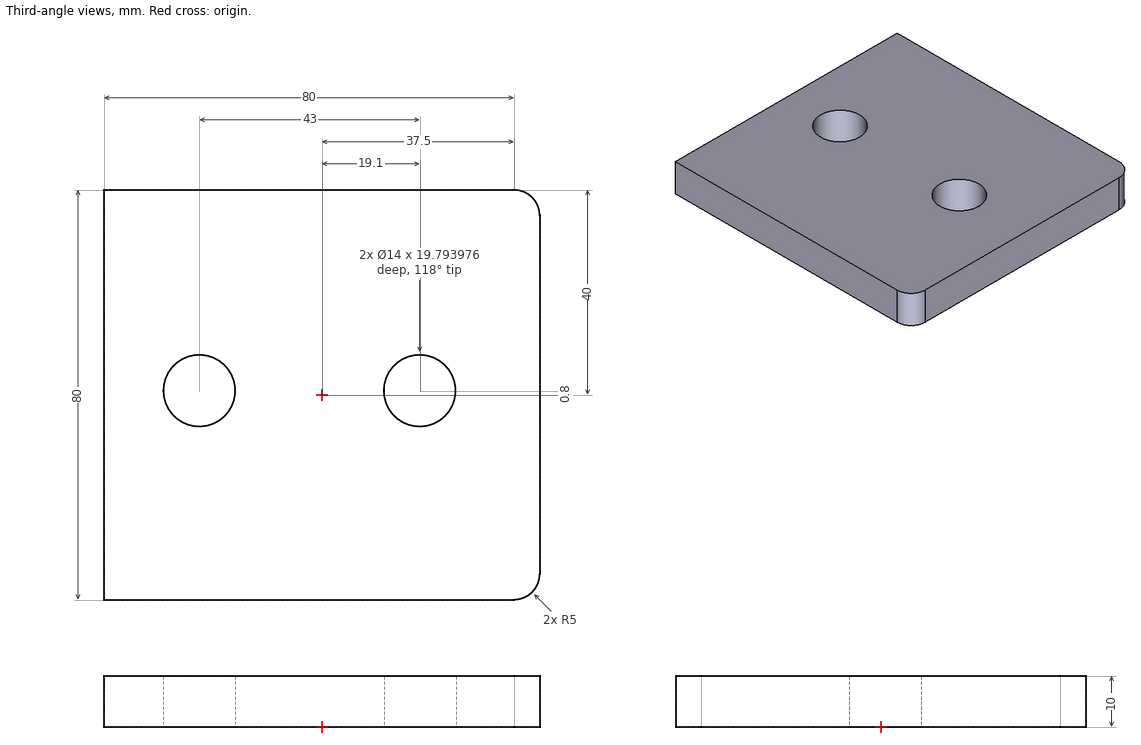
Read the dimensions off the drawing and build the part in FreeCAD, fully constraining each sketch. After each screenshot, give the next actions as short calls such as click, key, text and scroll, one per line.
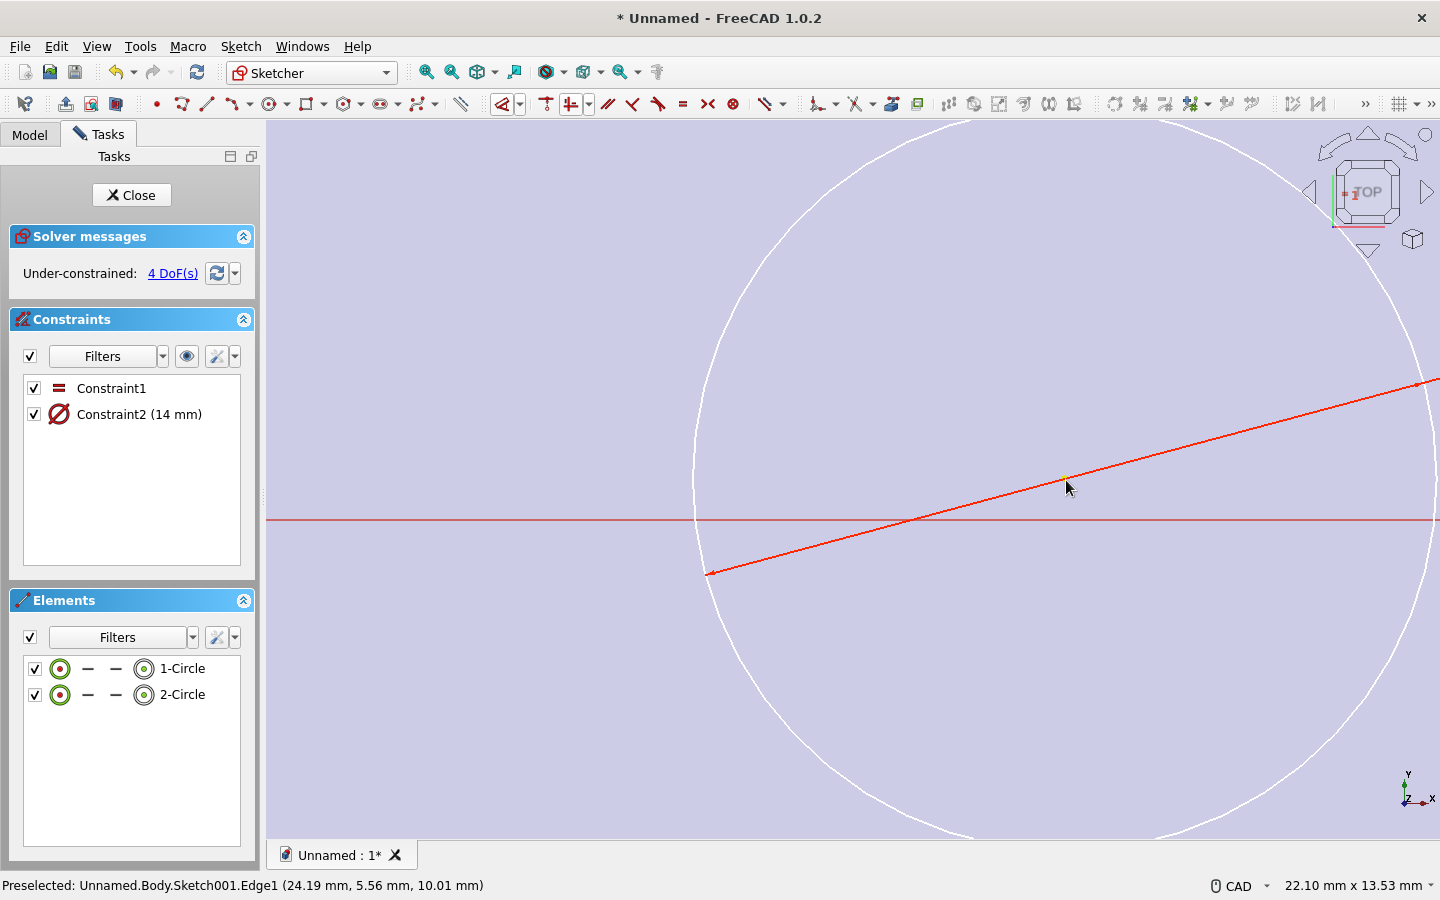
click(1065, 479)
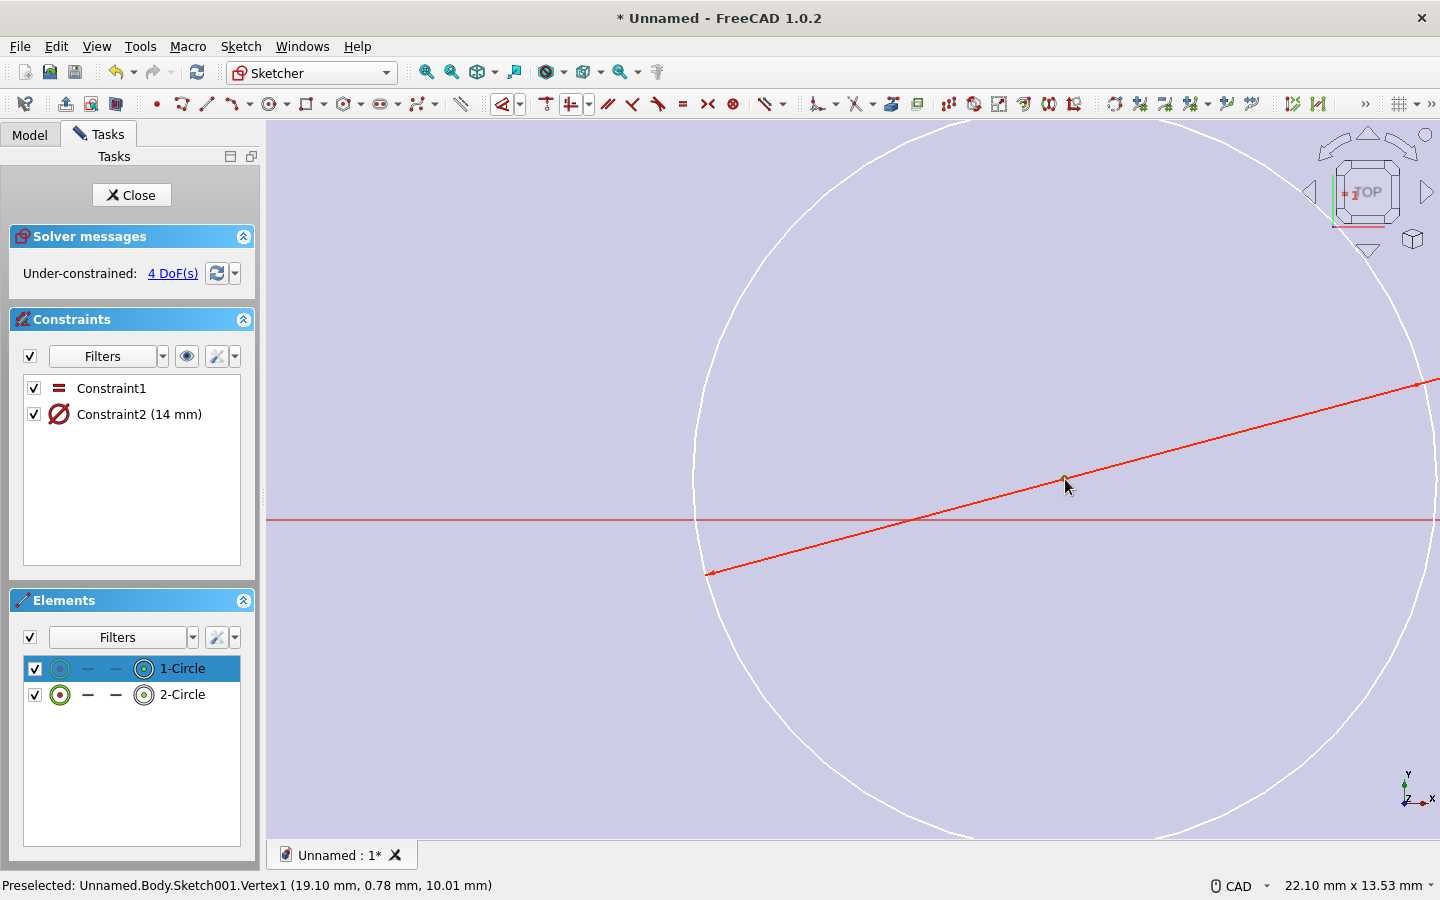
key(i)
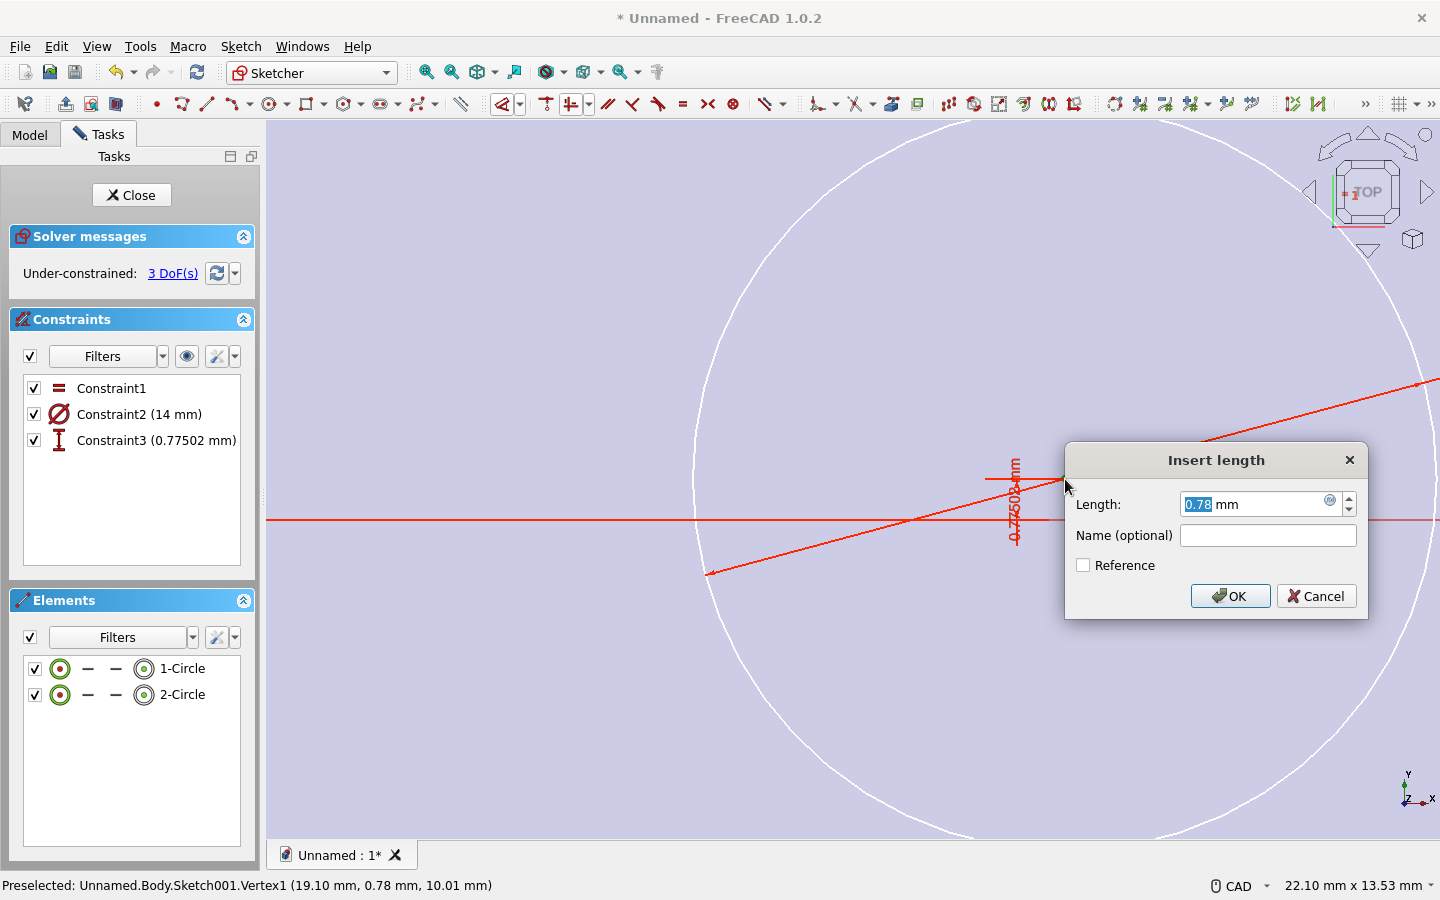
text(0.8)
key(Return)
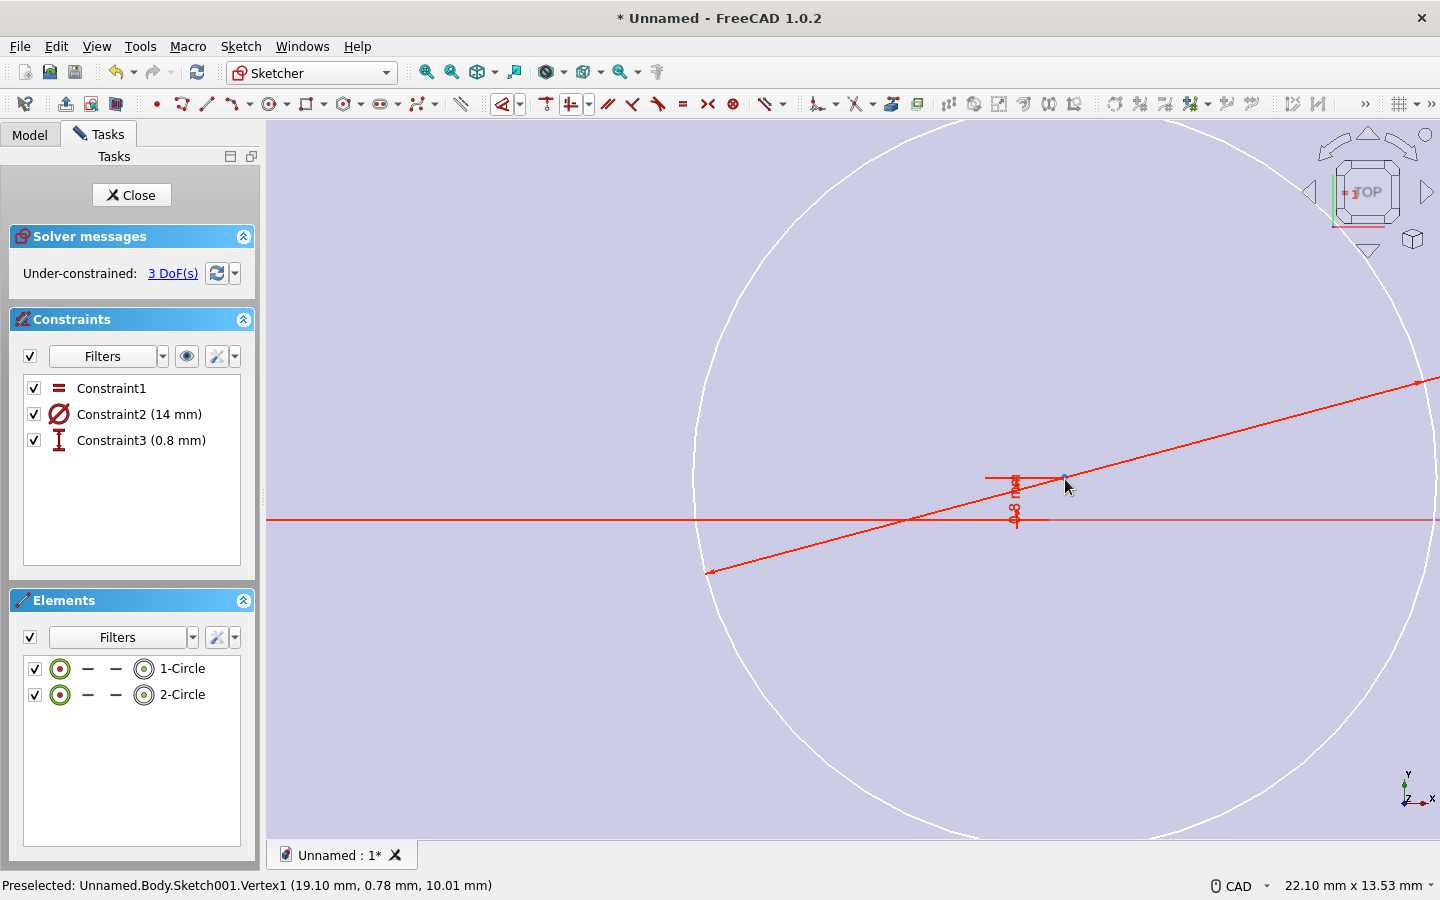
scroll(1067, 480, down, 7)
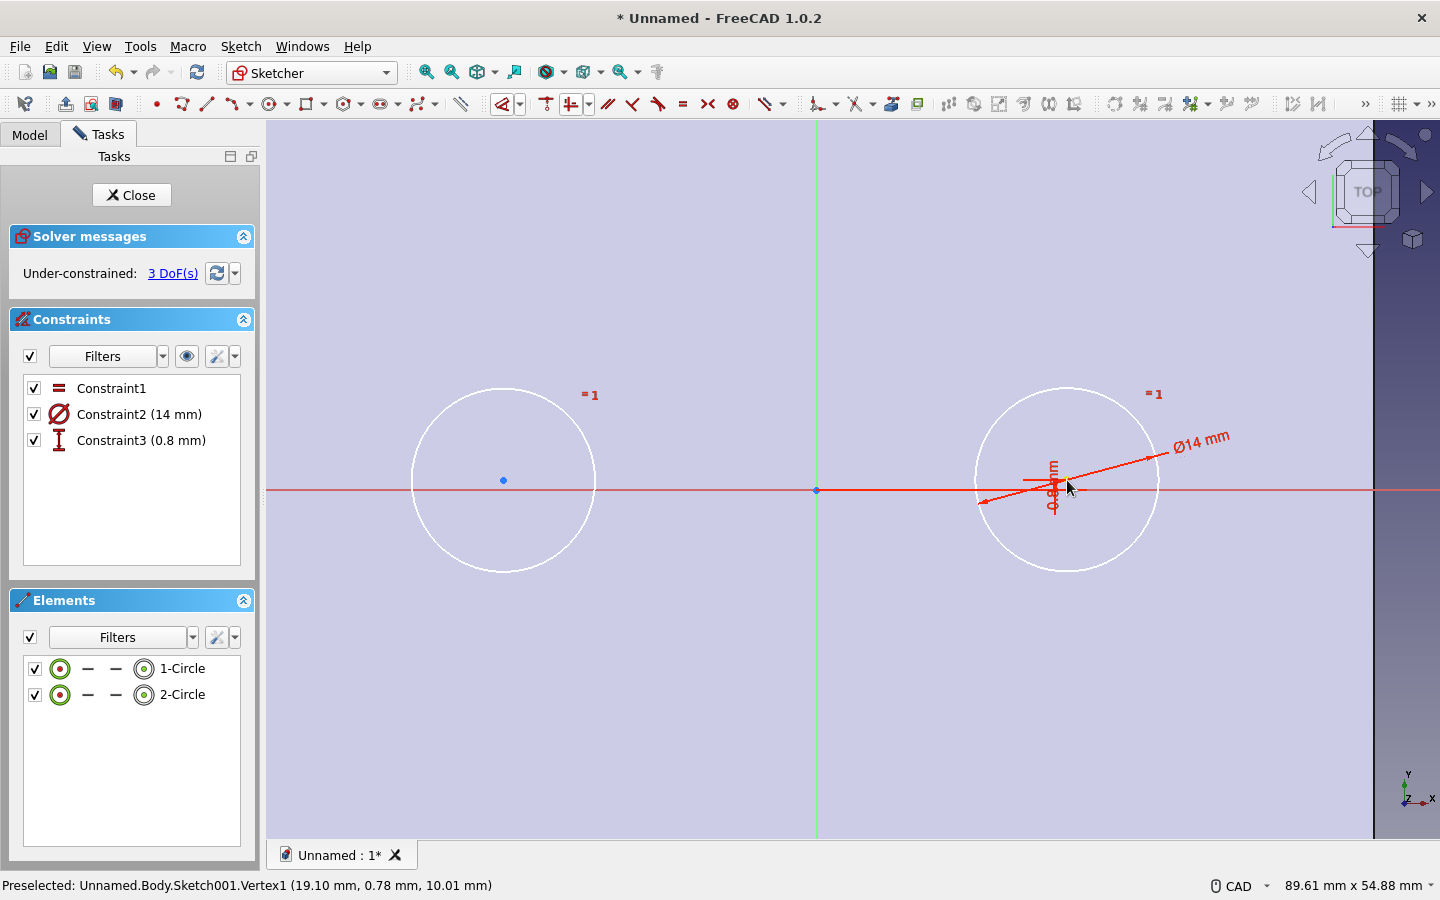
scroll(503, 480, up, 7)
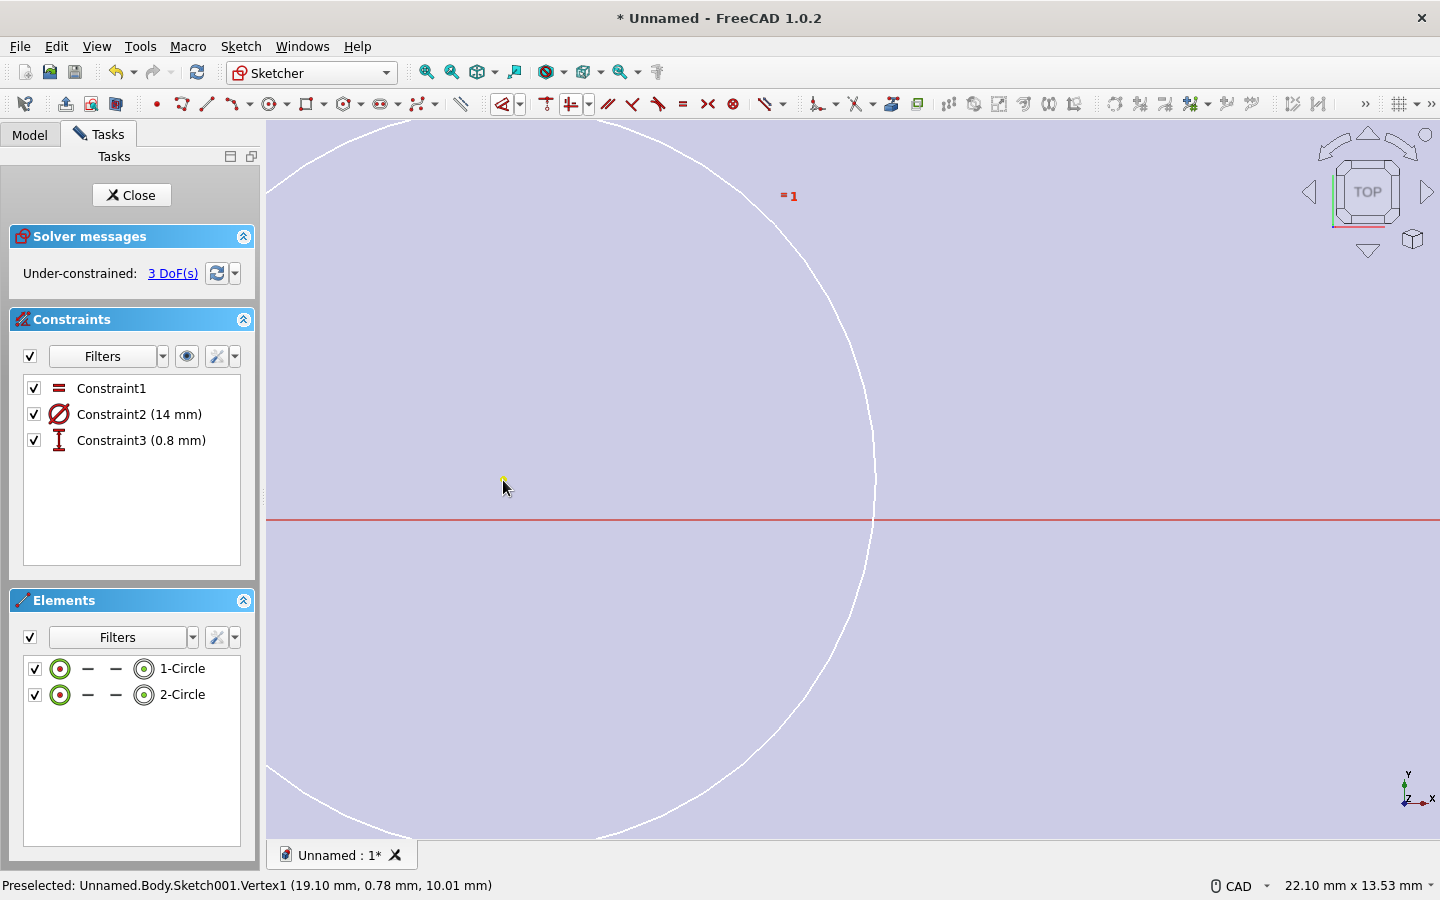
click(504, 479)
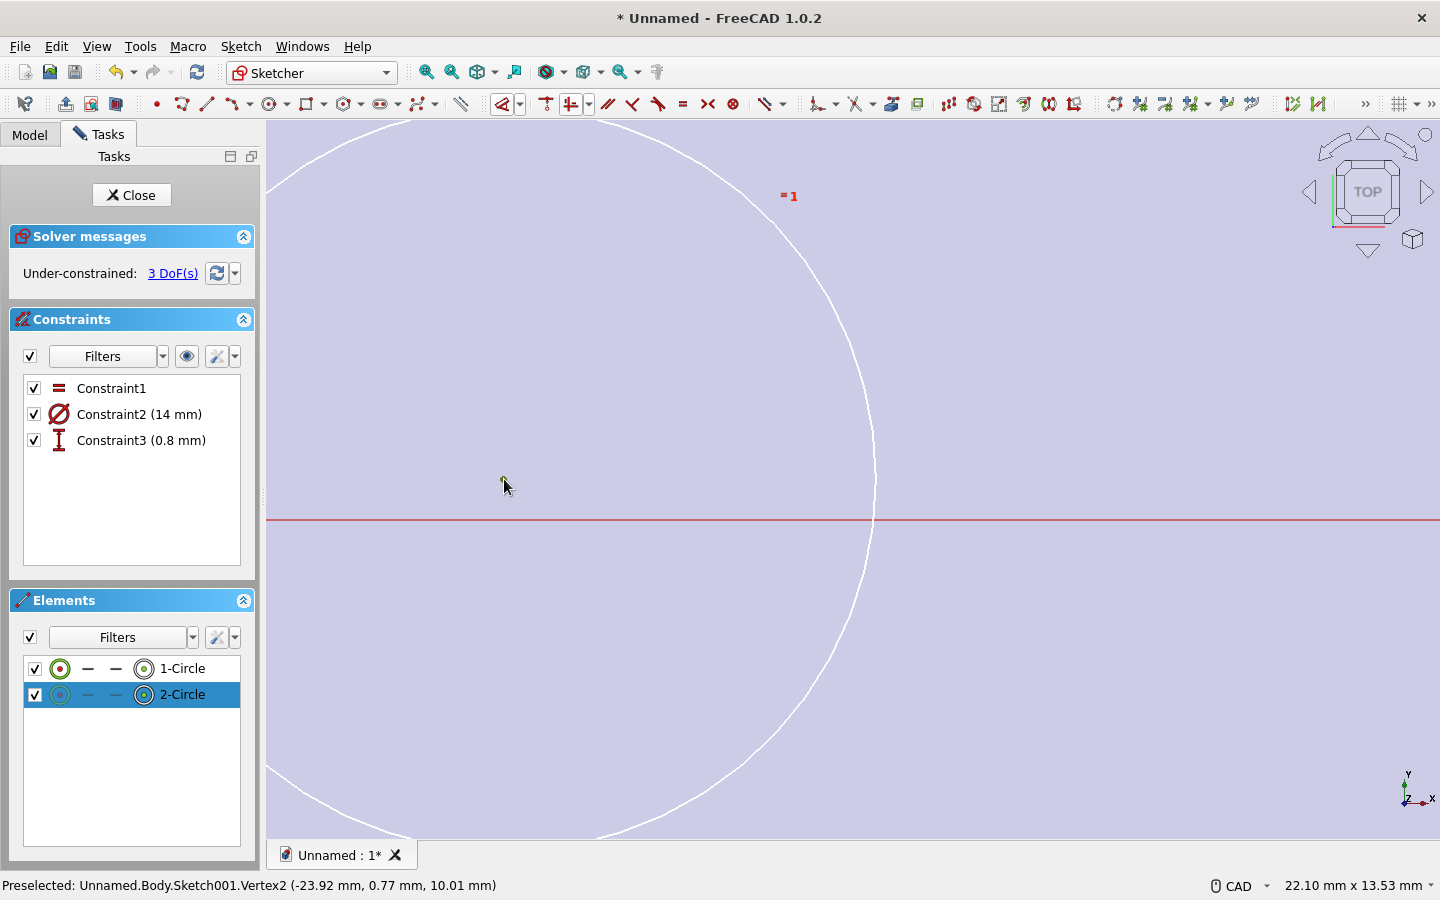
key(i)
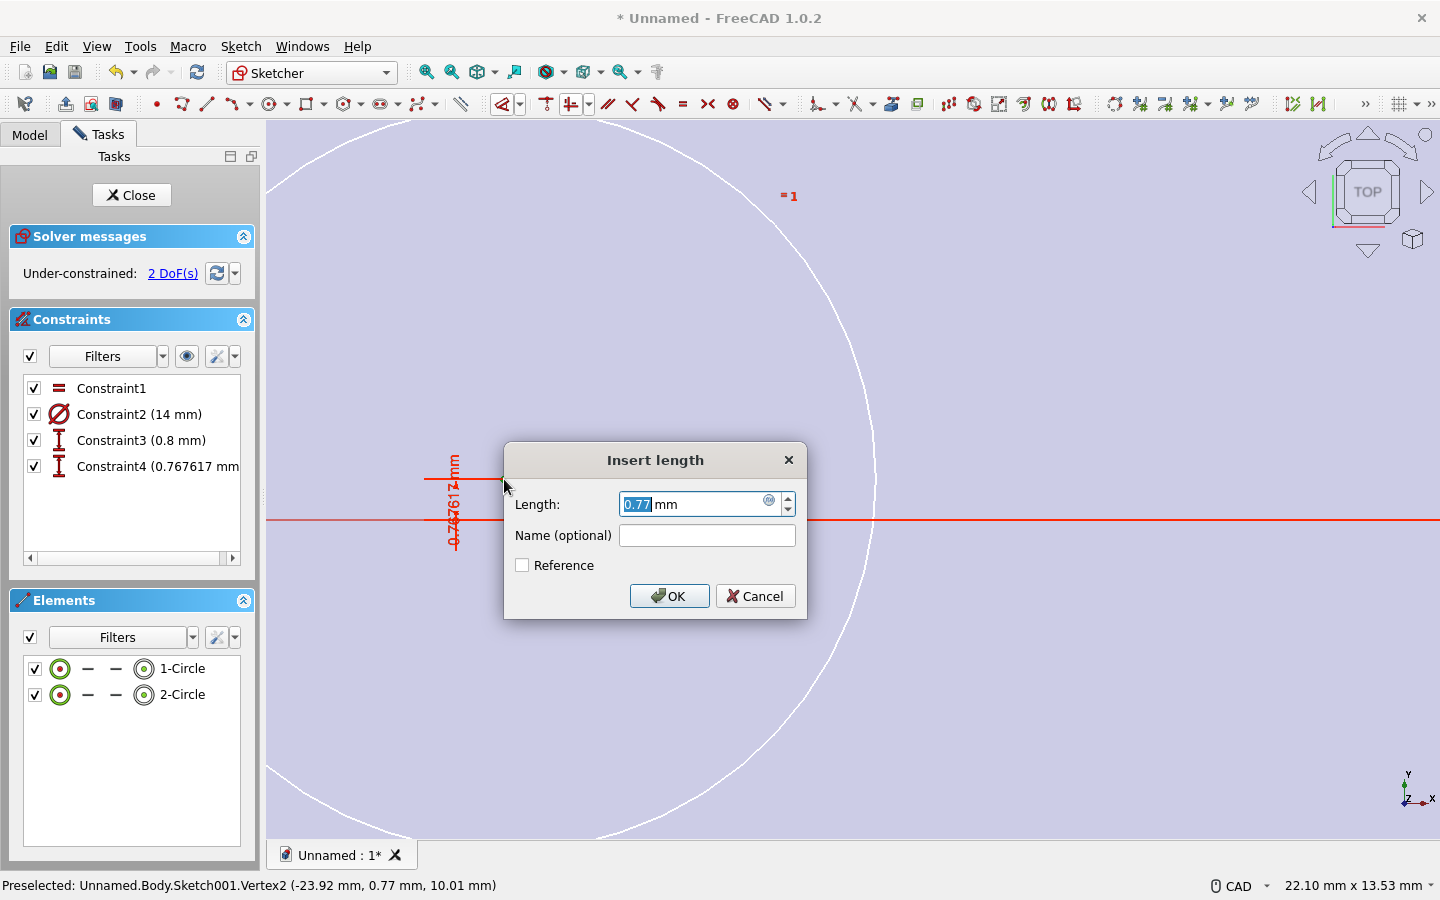
text(0.8)
key(Return)